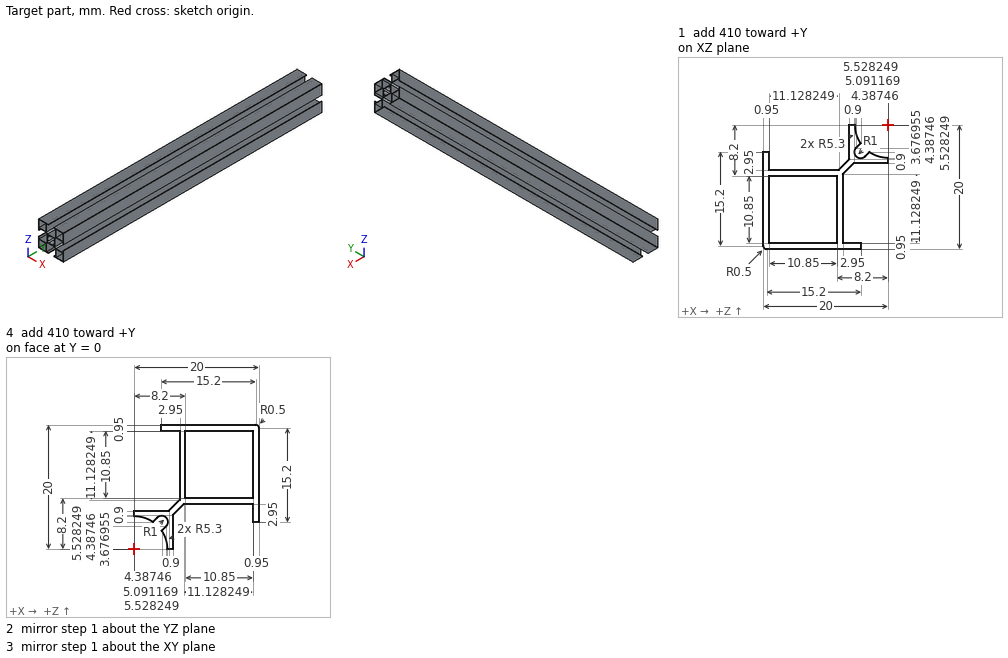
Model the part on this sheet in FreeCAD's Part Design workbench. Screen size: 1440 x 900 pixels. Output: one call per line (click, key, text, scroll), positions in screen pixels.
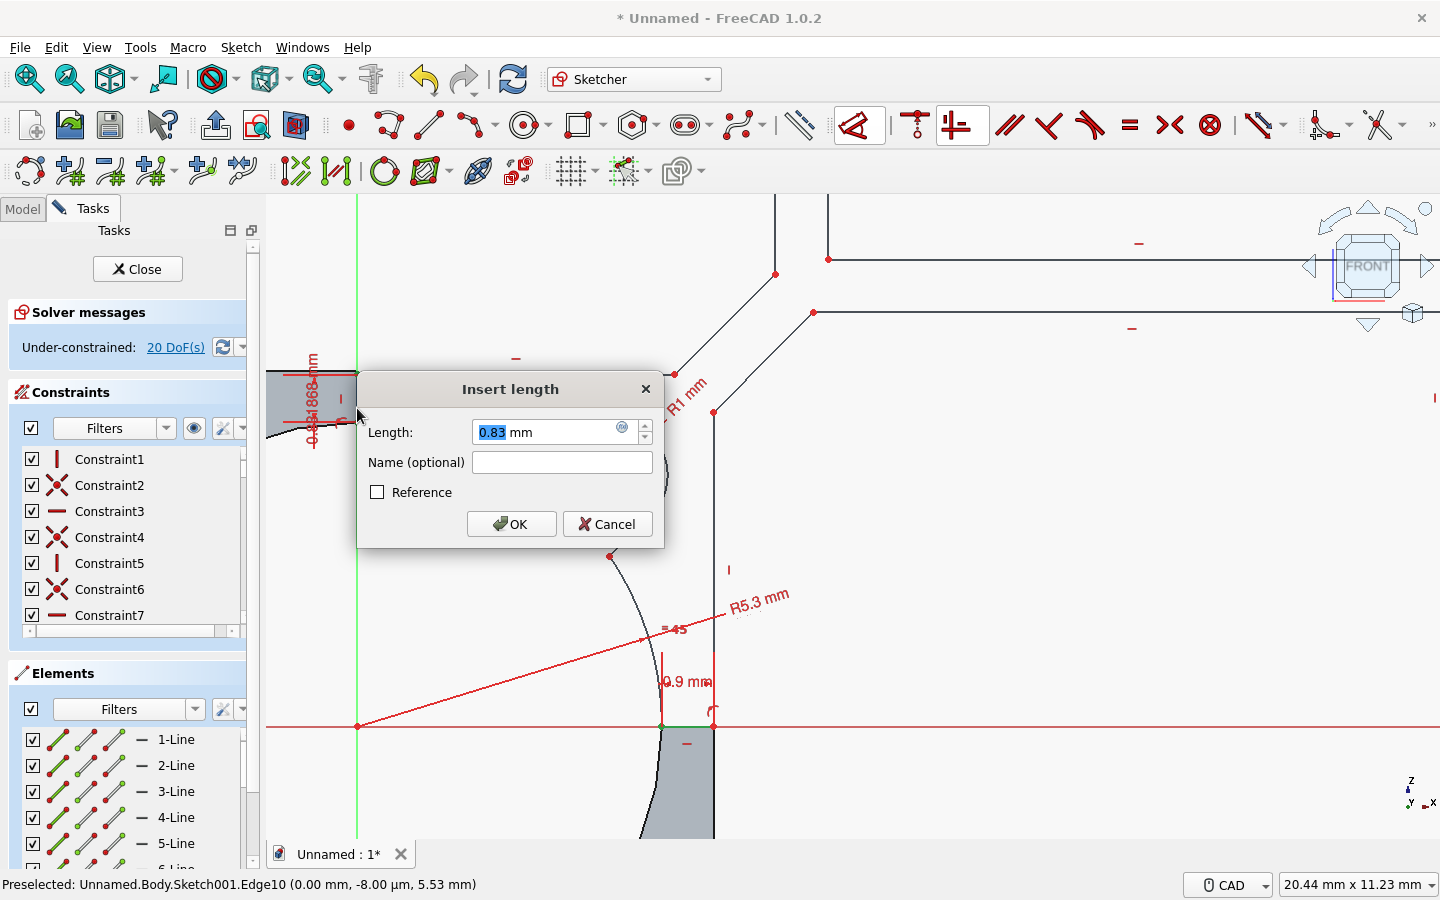
text(0.9)
key(Return)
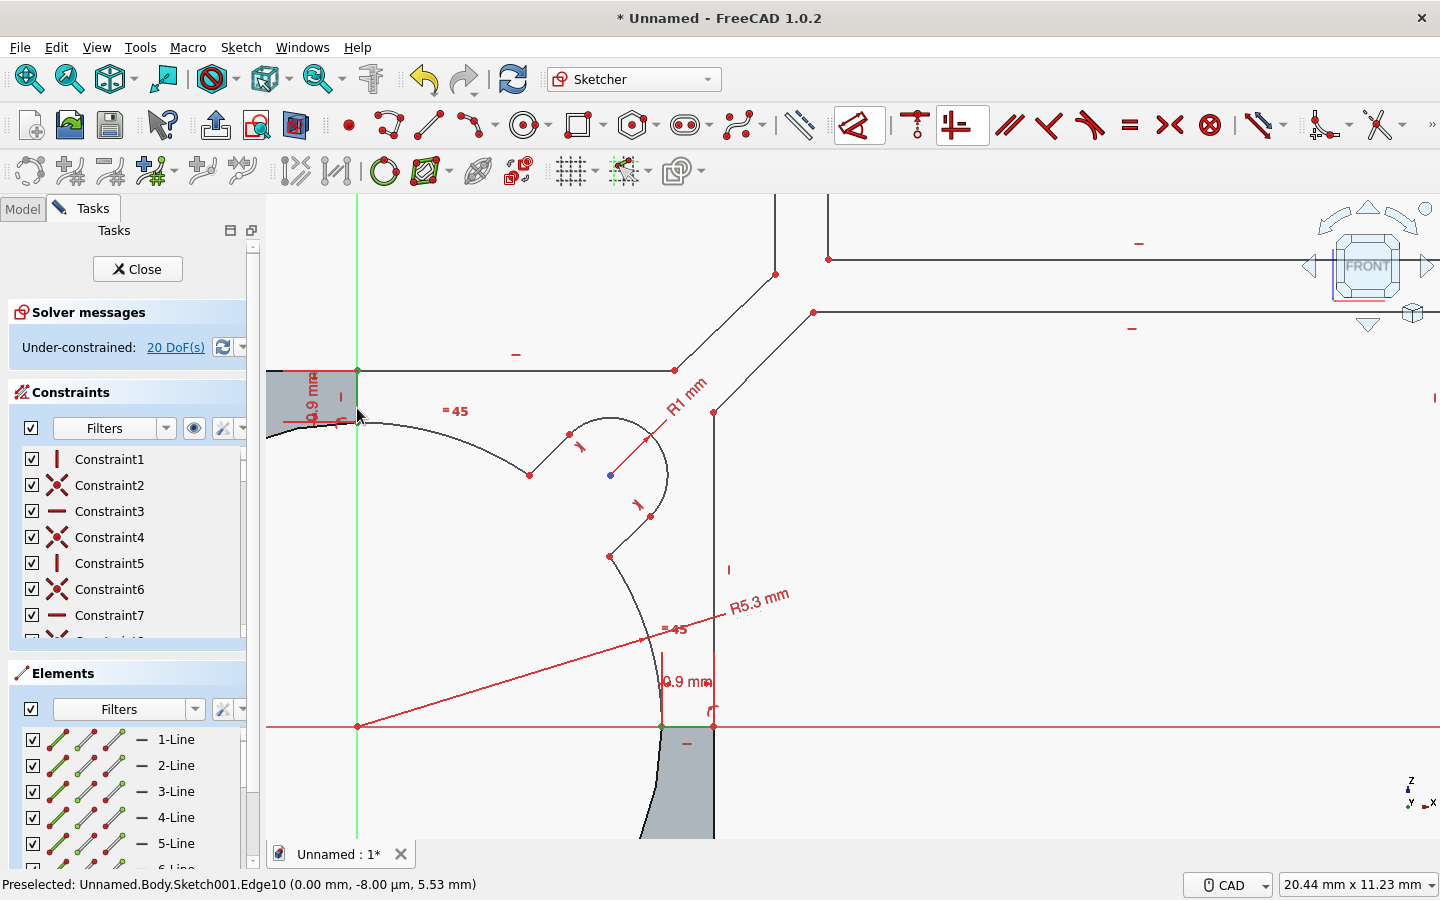
scroll(699, 728, down, 5)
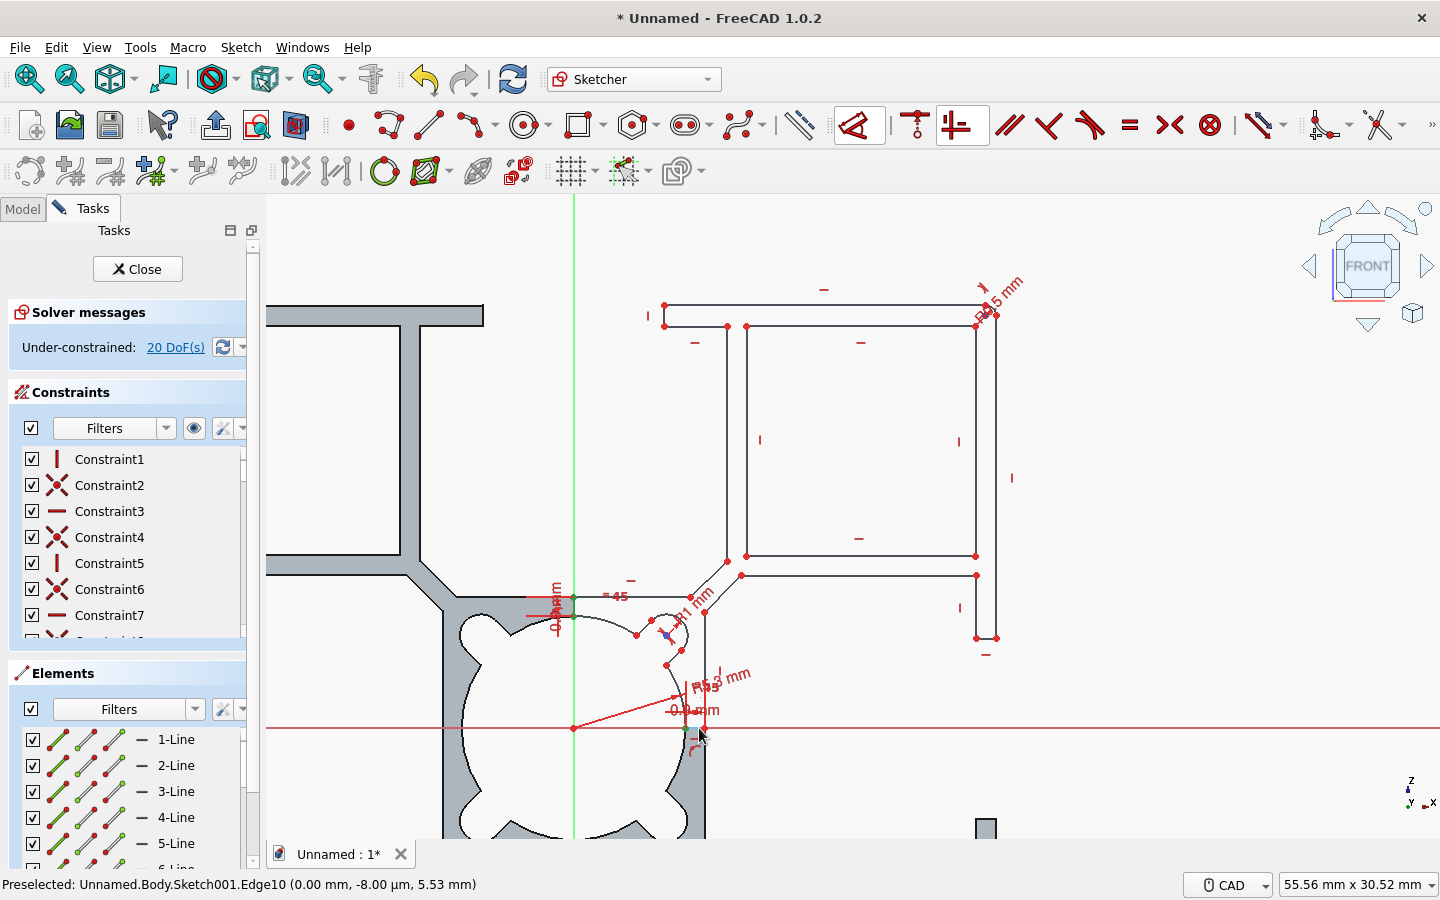
click(996, 316)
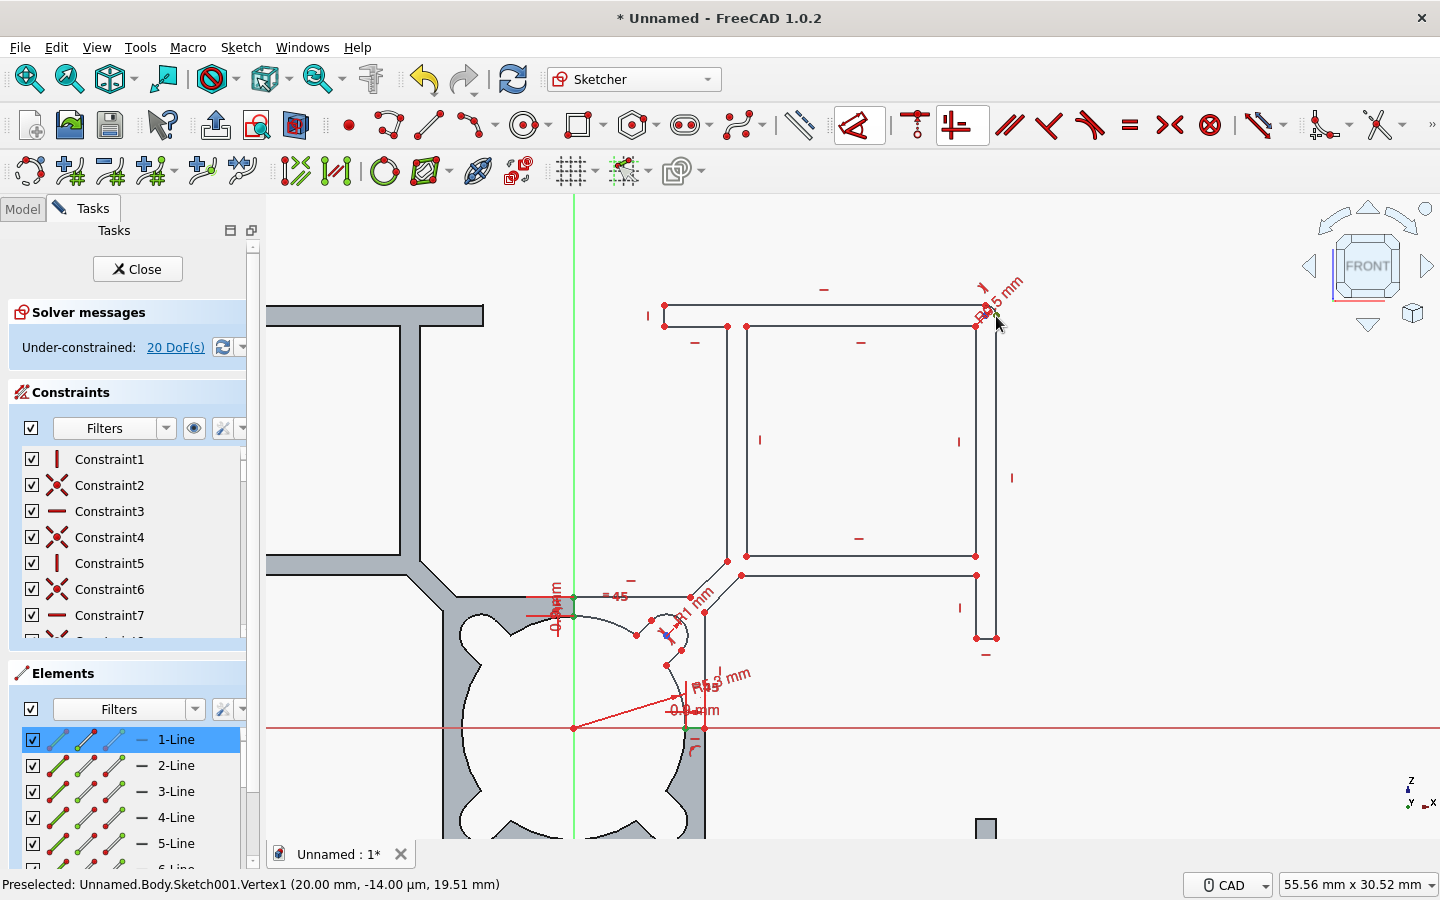
click(880, 126)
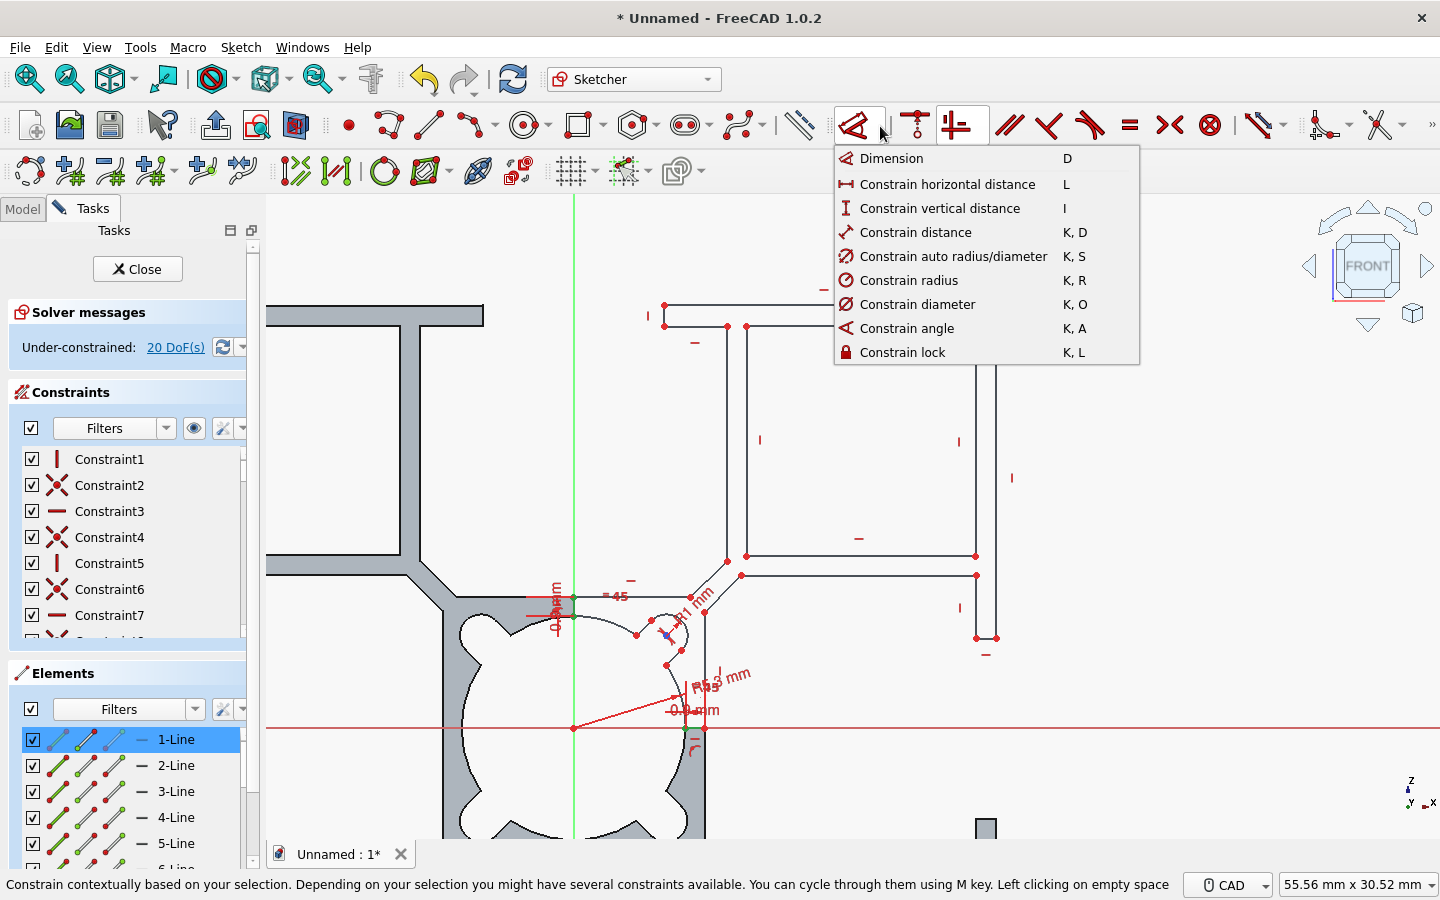
click(987, 184)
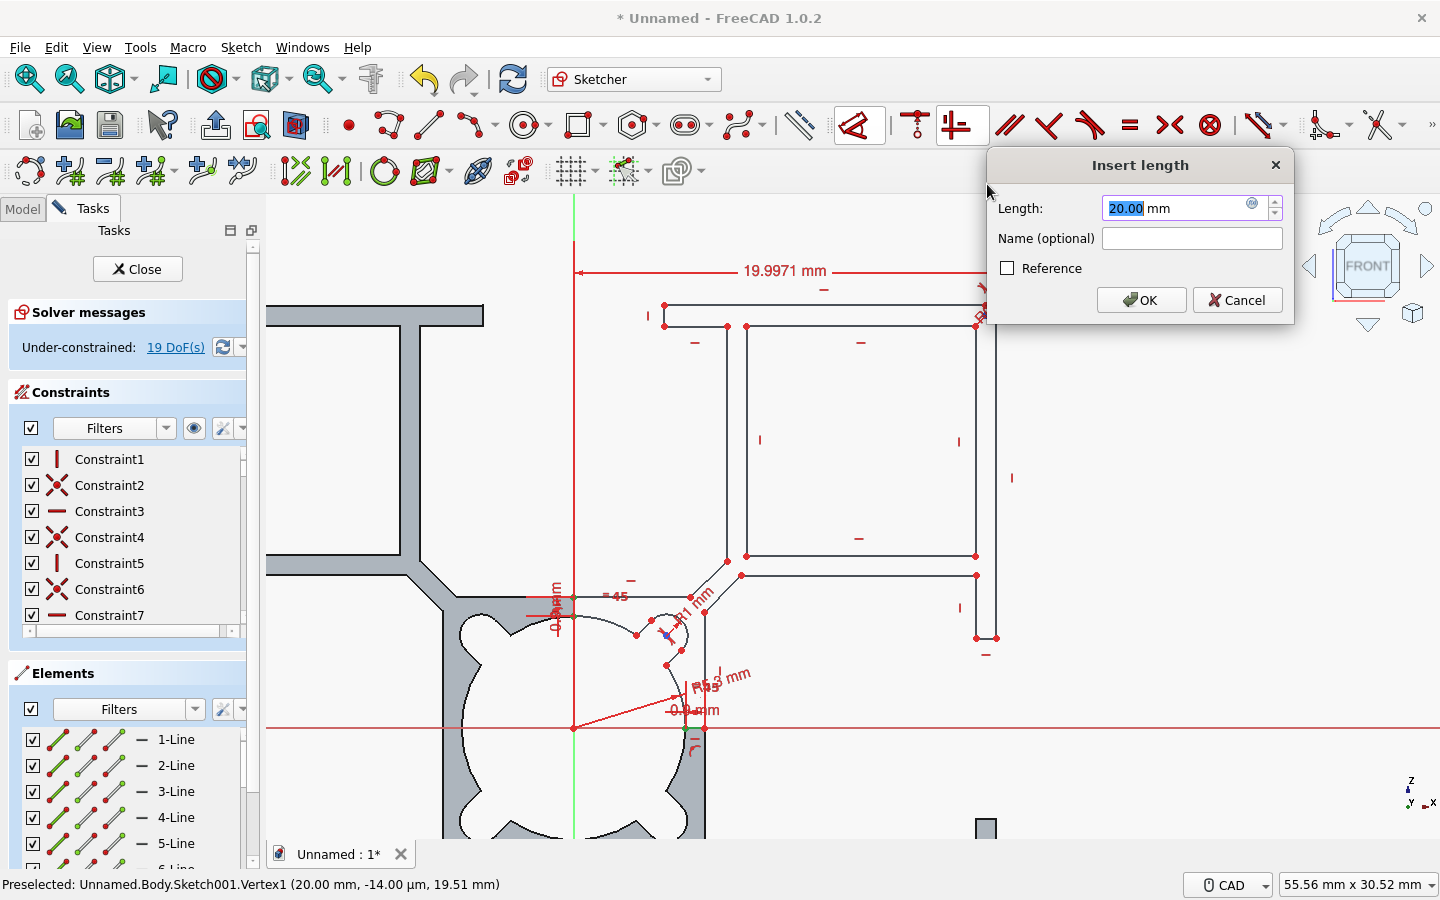
text(20)
key(Return)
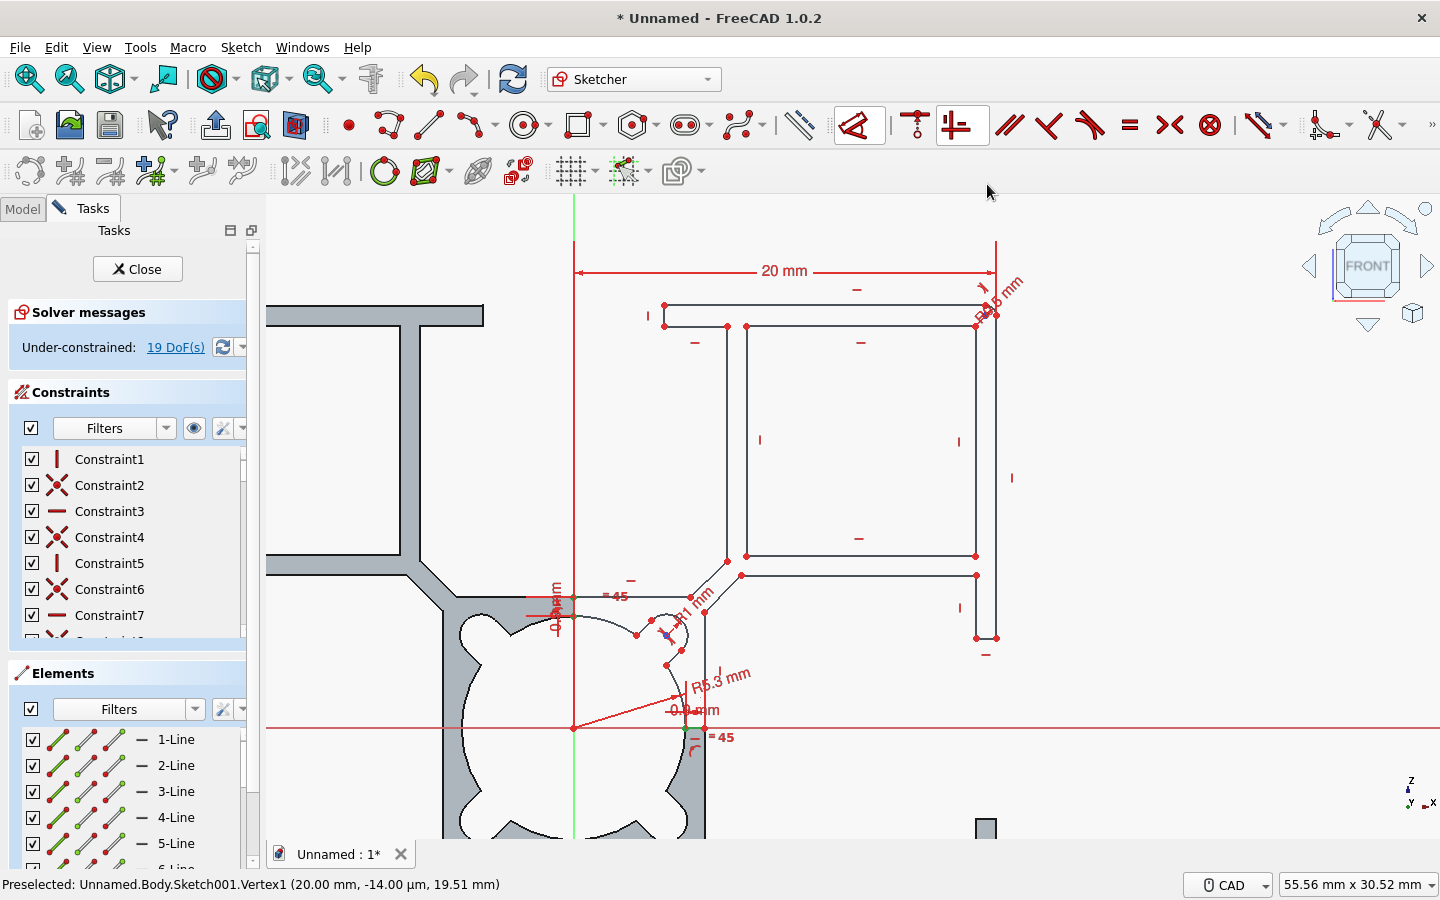
click(664, 305)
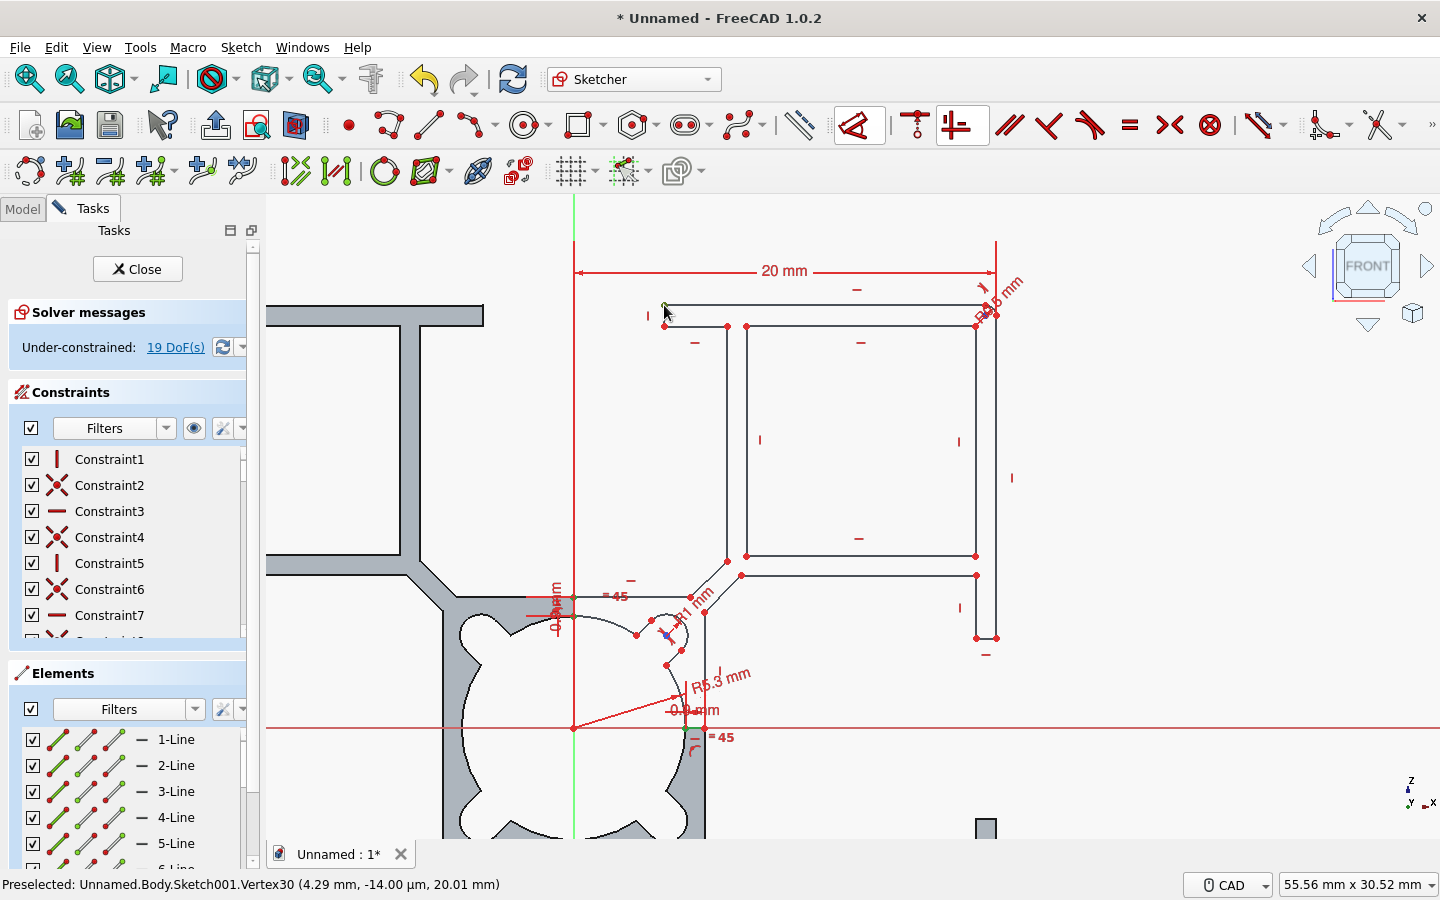
key(i)